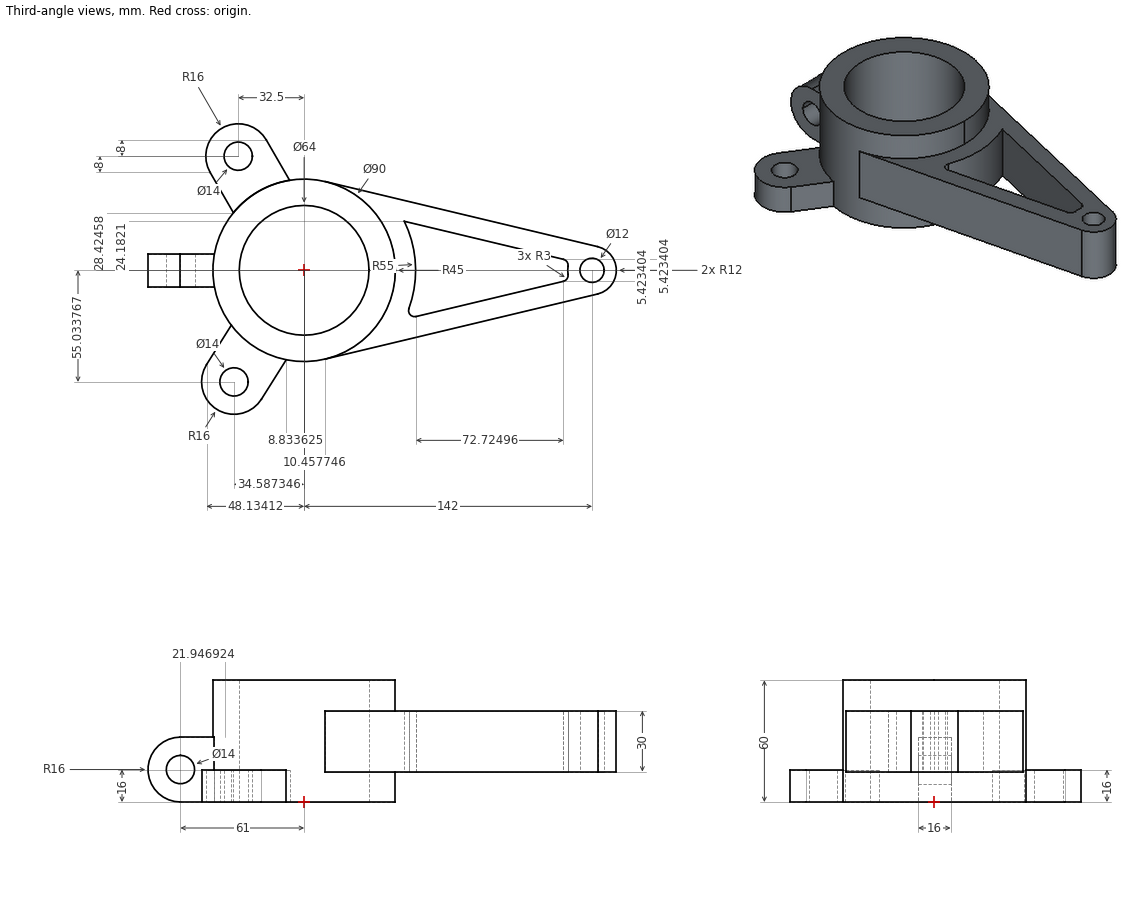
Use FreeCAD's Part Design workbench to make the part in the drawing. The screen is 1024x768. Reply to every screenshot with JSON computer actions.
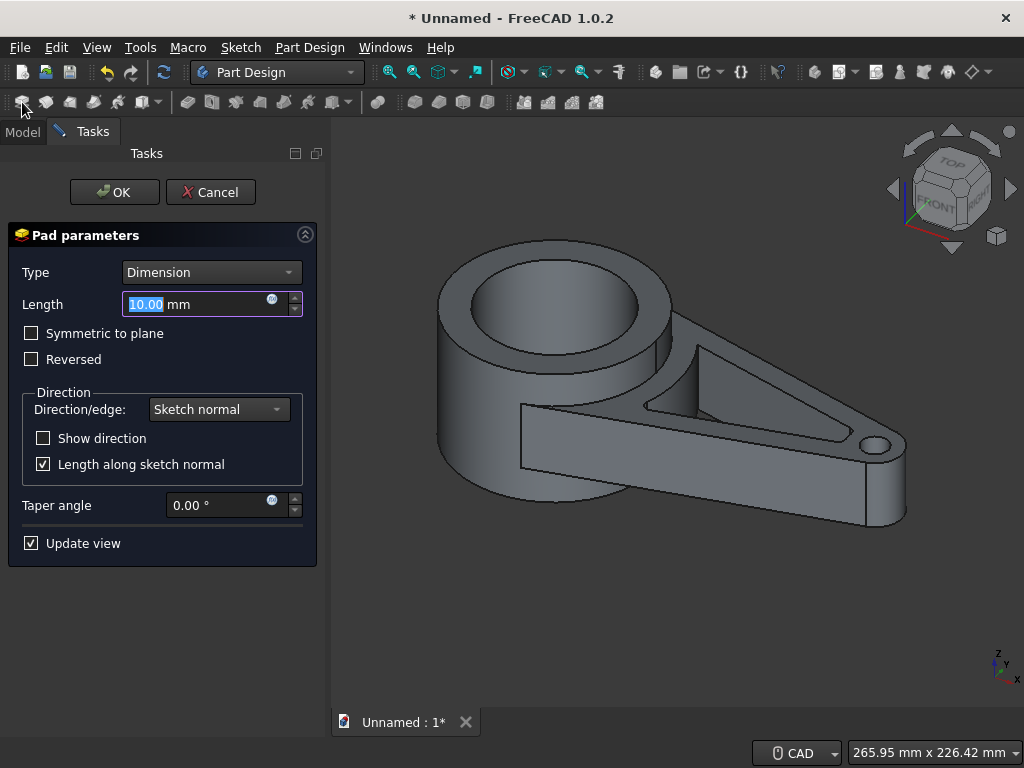
{"action": "type", "text": "16"}
{"action": "key", "text": "Tab"}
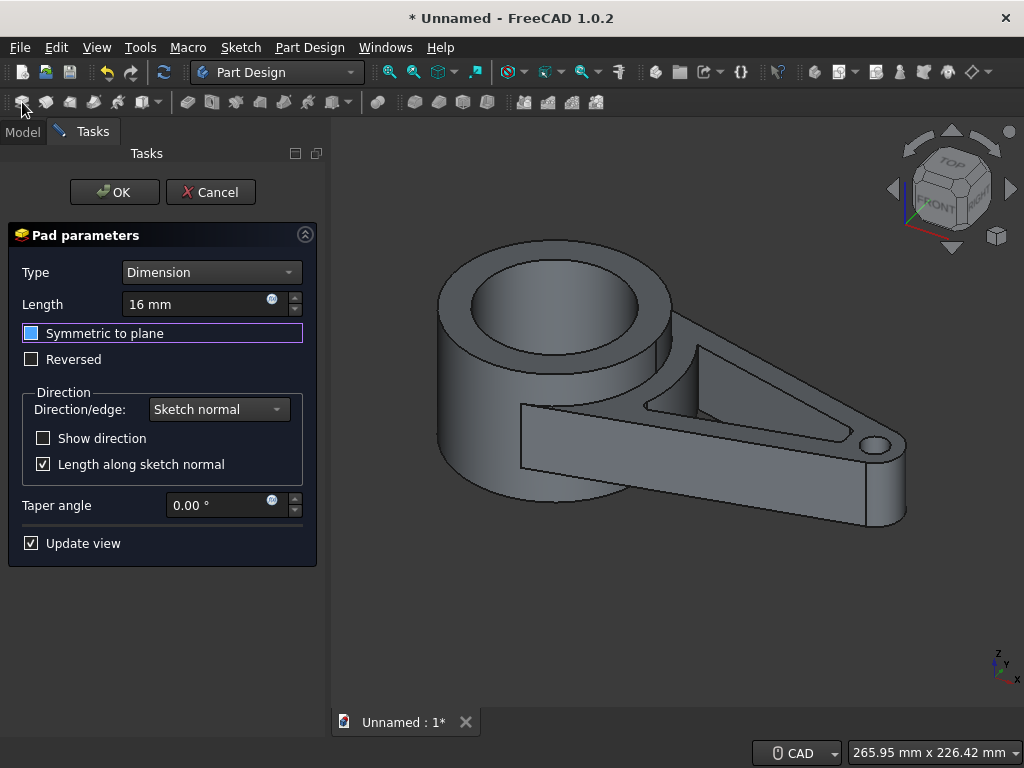
{"action": "left_click", "coordinate": [115, 192]}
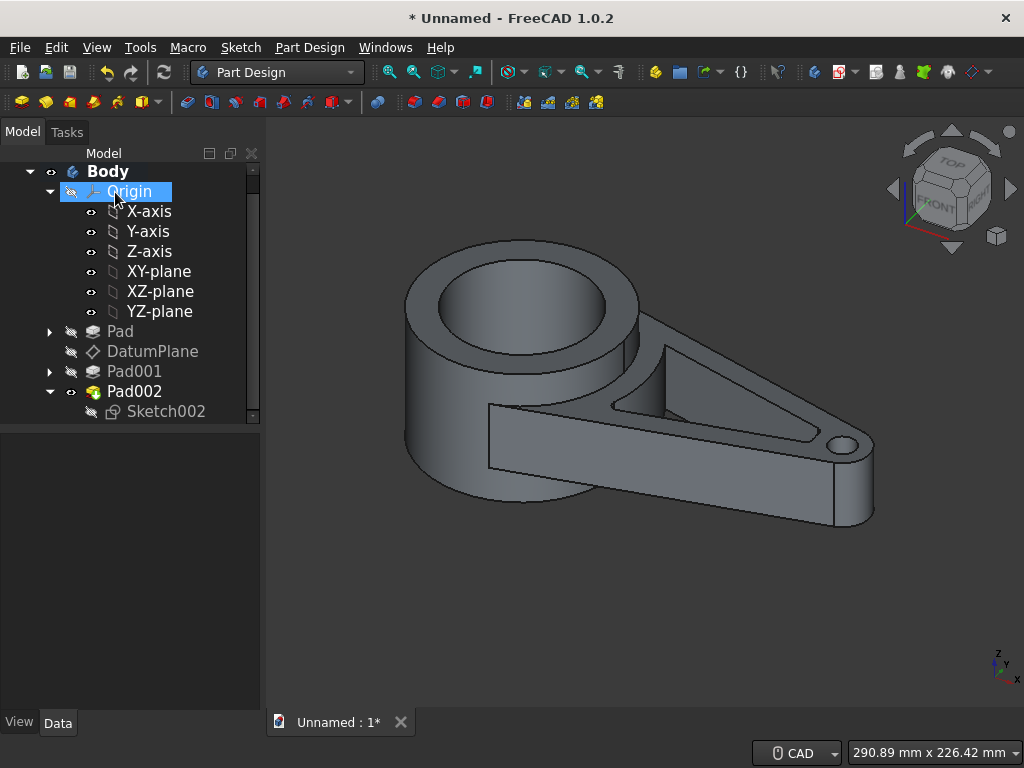
{"action": "key", "text": "5"}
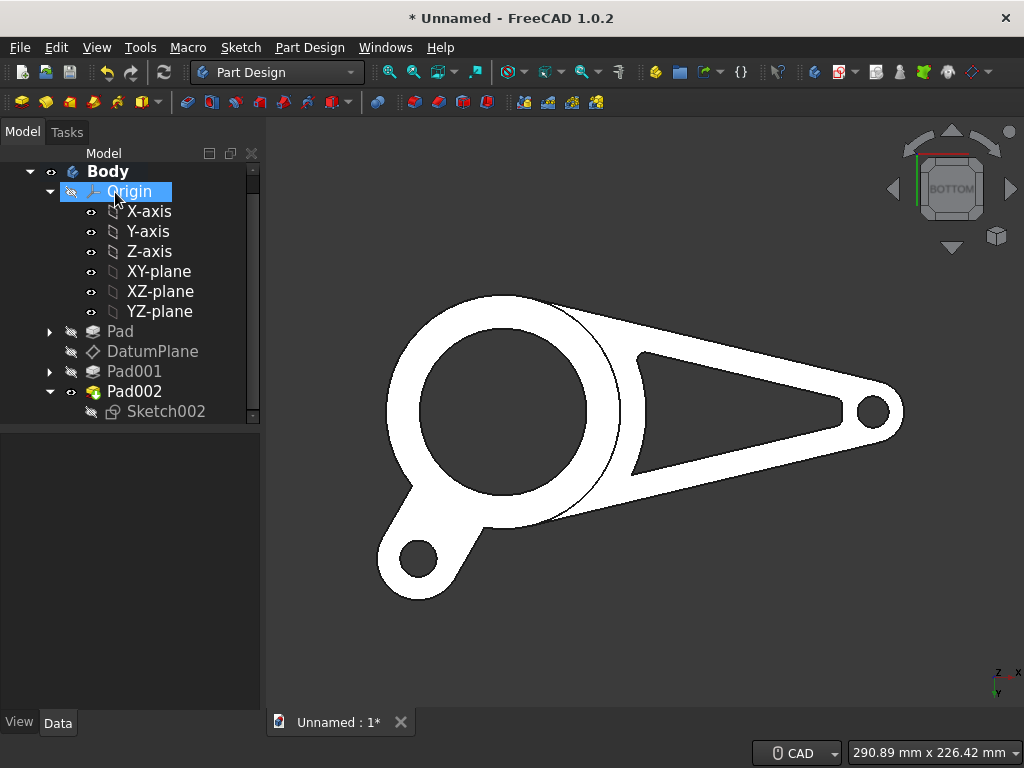
{"action": "left_click", "coordinate": [429, 490]}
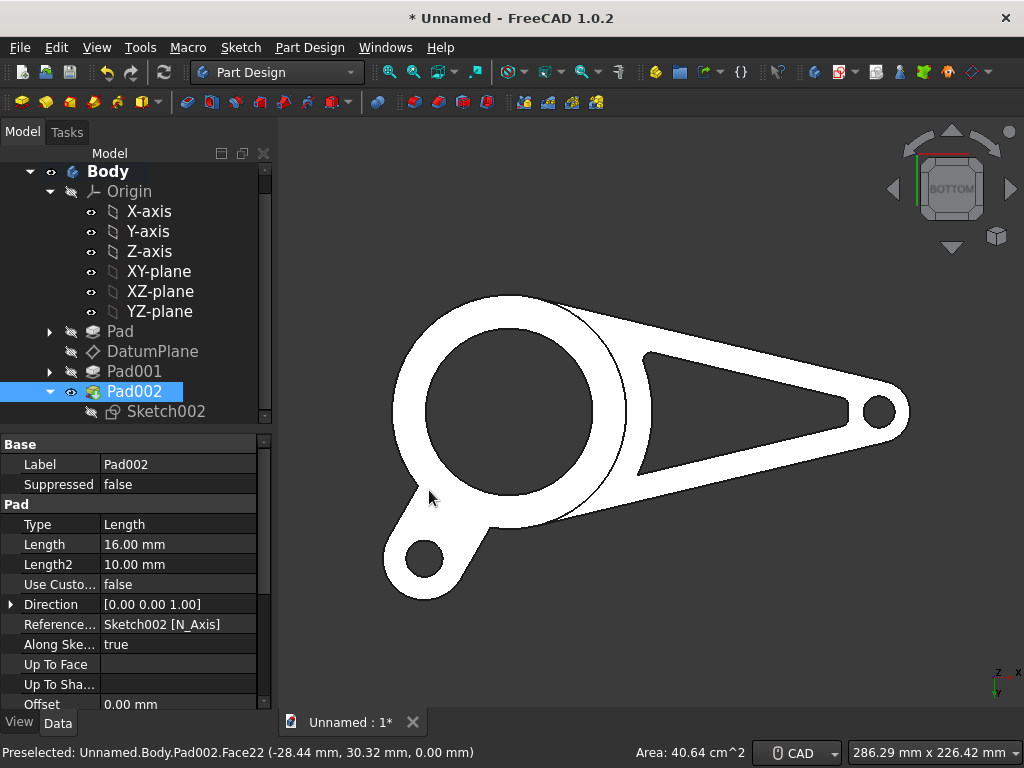
{"action": "left_click", "coordinate": [840, 72]}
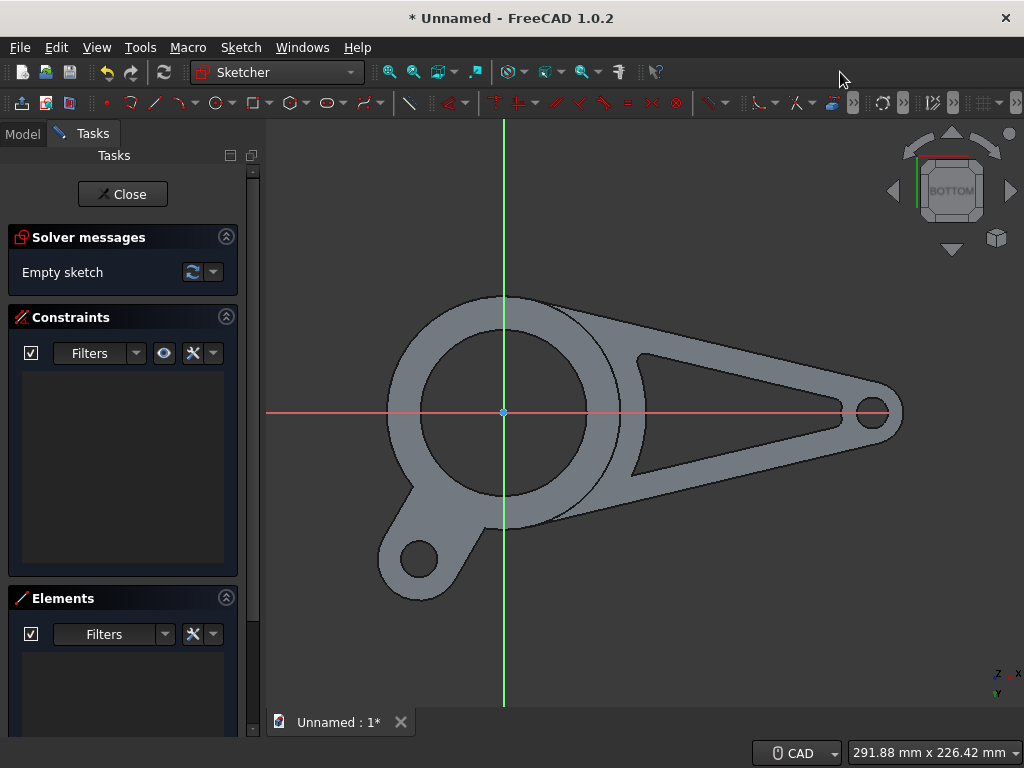
{"action": "scroll", "coordinate": [331, 251], "scroll_direction": "up", "scroll_amount": 4}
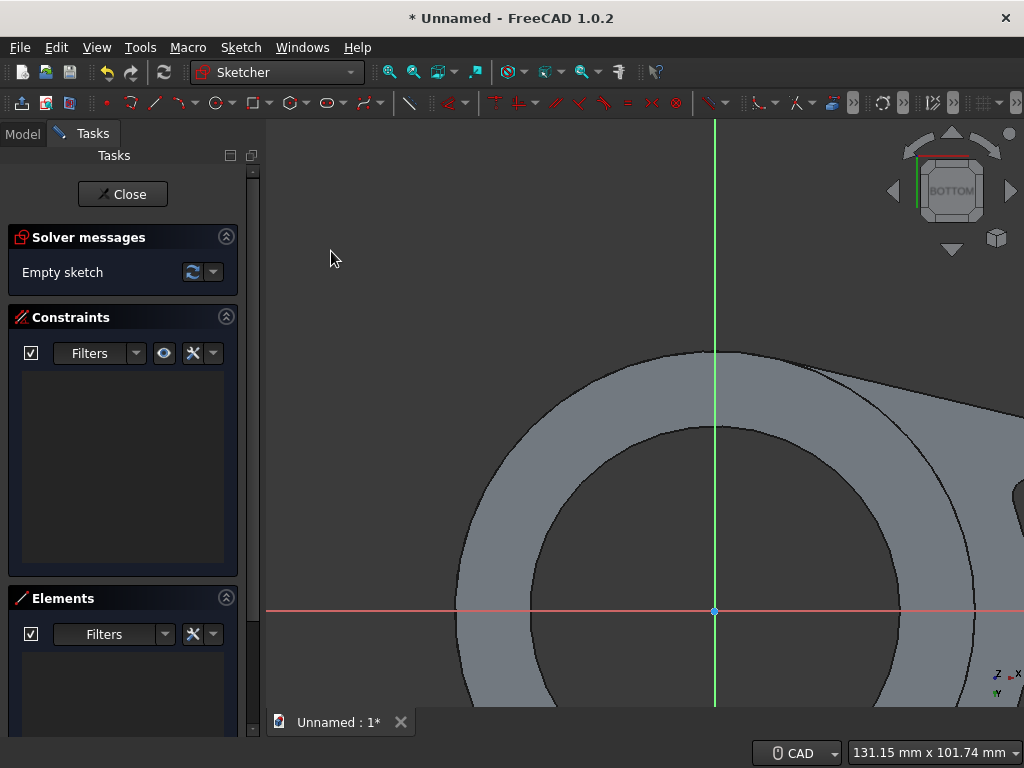
{"action": "key", "text": "g l"}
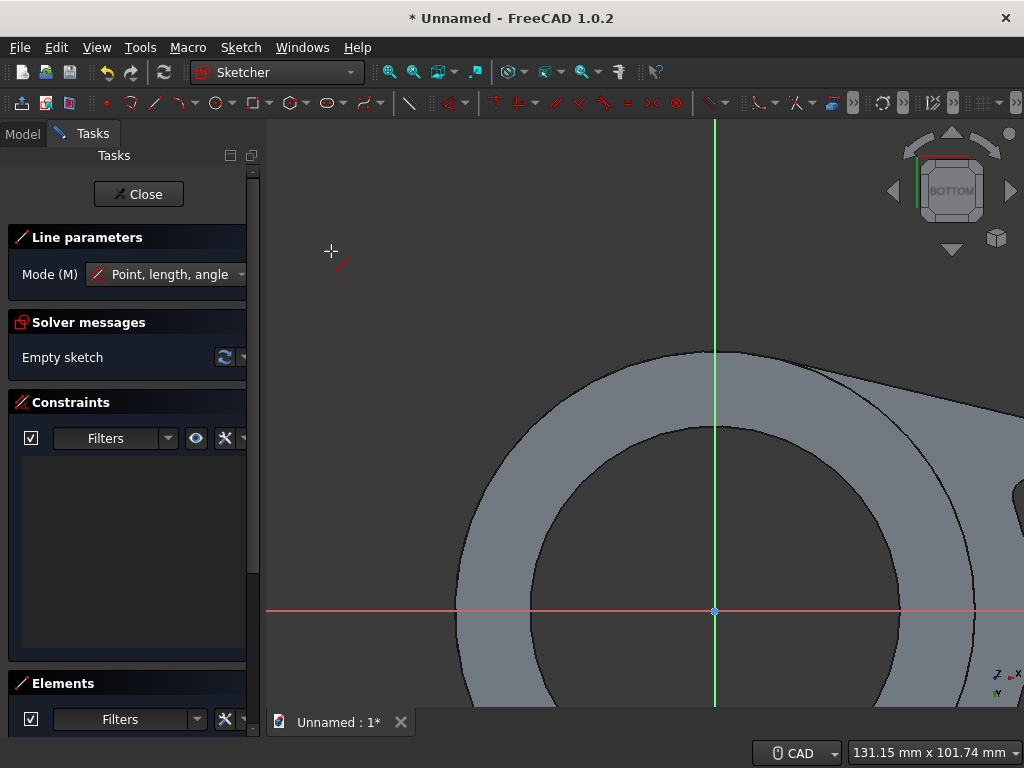
{"action": "left_click", "coordinate": [507, 455]}
{"action": "left_click", "coordinate": [437, 342]}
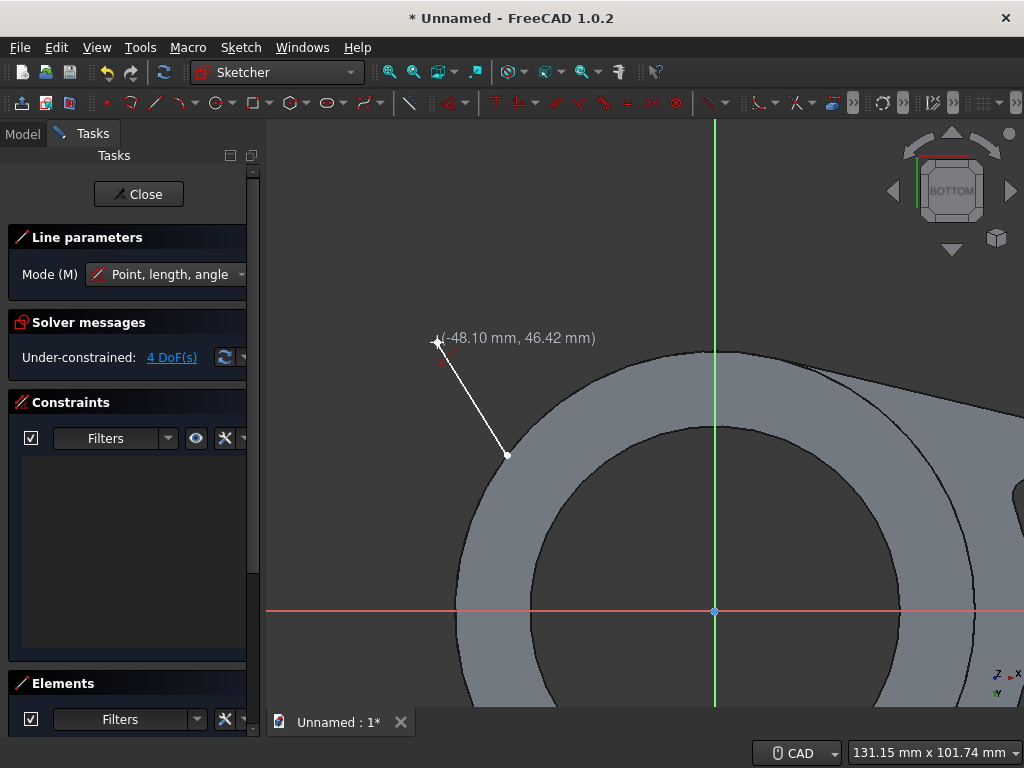
{"action": "left_click", "coordinate": [593, 244]}
{"action": "left_click", "coordinate": [664, 356]}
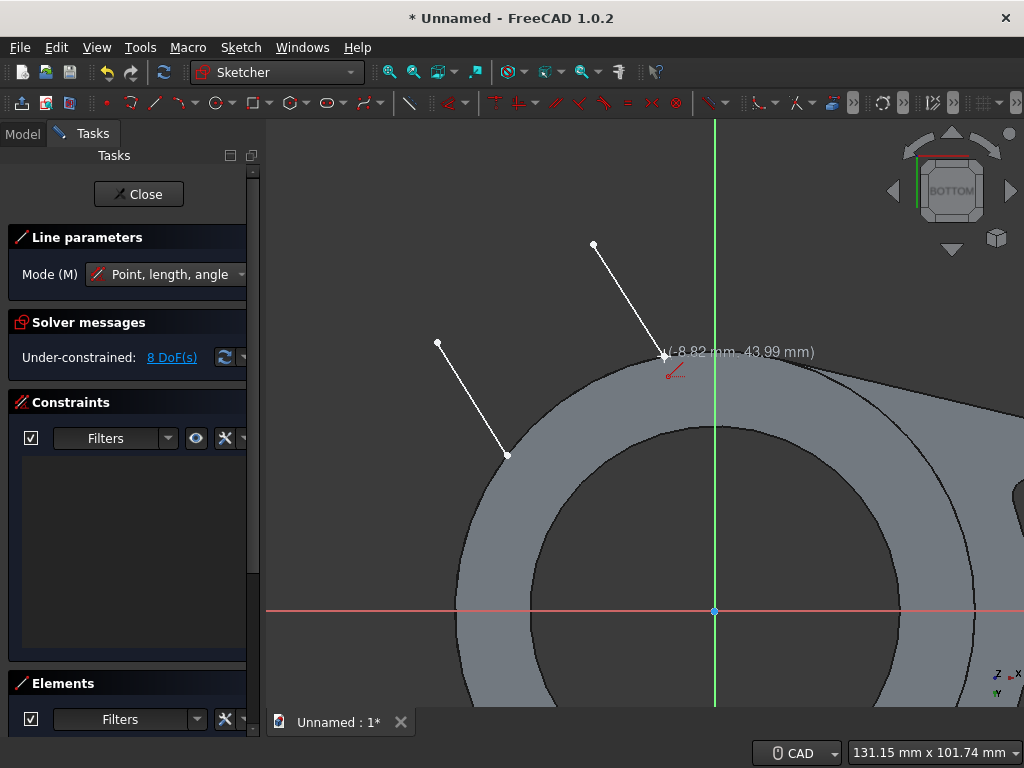
{"action": "key", "text": "g 3 a"}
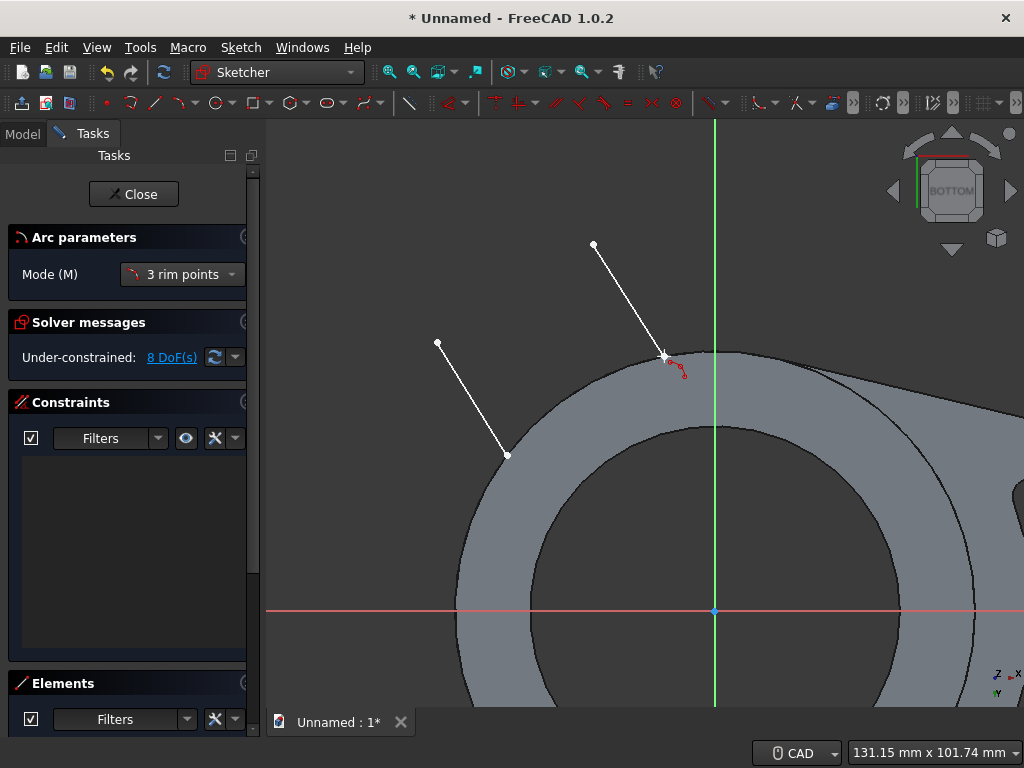
{"action": "left_click", "coordinate": [437, 343]}
{"action": "left_click", "coordinate": [593, 245]}
{"action": "left_click", "coordinate": [466, 215]}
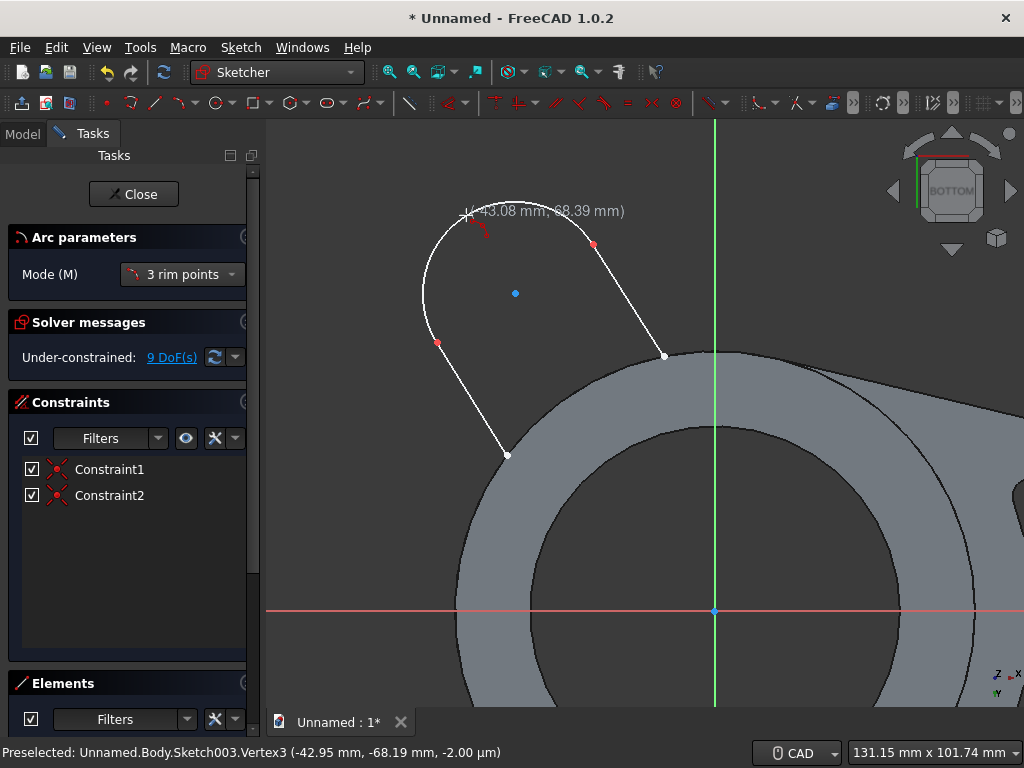
{"action": "left_click", "coordinate": [664, 357]}
{"action": "left_click", "coordinate": [507, 456]}
{"action": "left_click", "coordinate": [577, 391]}